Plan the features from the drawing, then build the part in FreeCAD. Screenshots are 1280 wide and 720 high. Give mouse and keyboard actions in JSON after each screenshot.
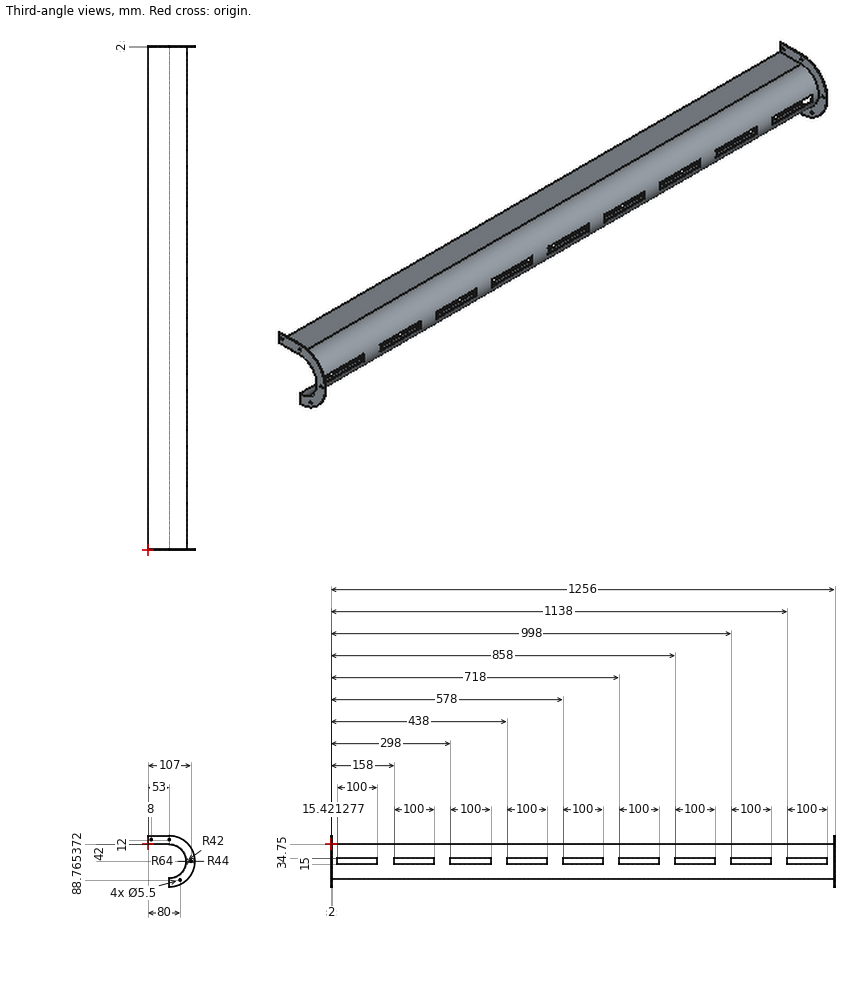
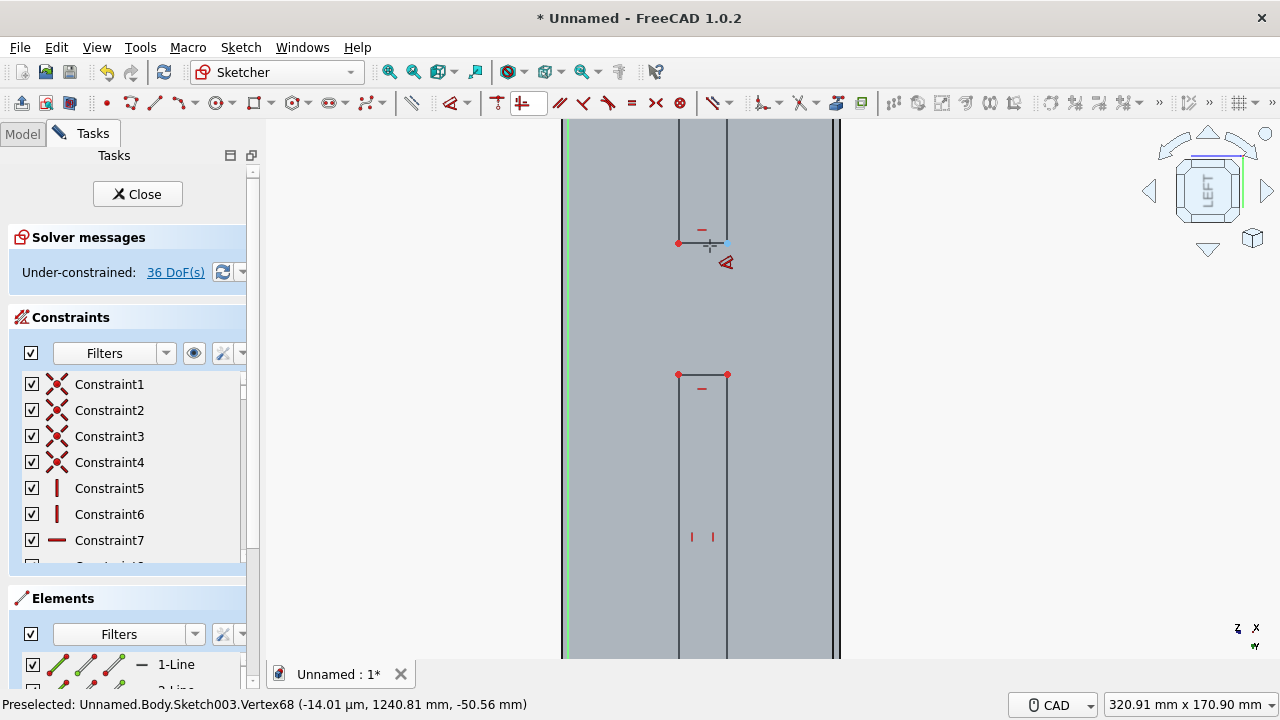
{"action": "left_click", "coordinate": [703, 243]}
{"action": "left_click", "coordinate": [703, 209]}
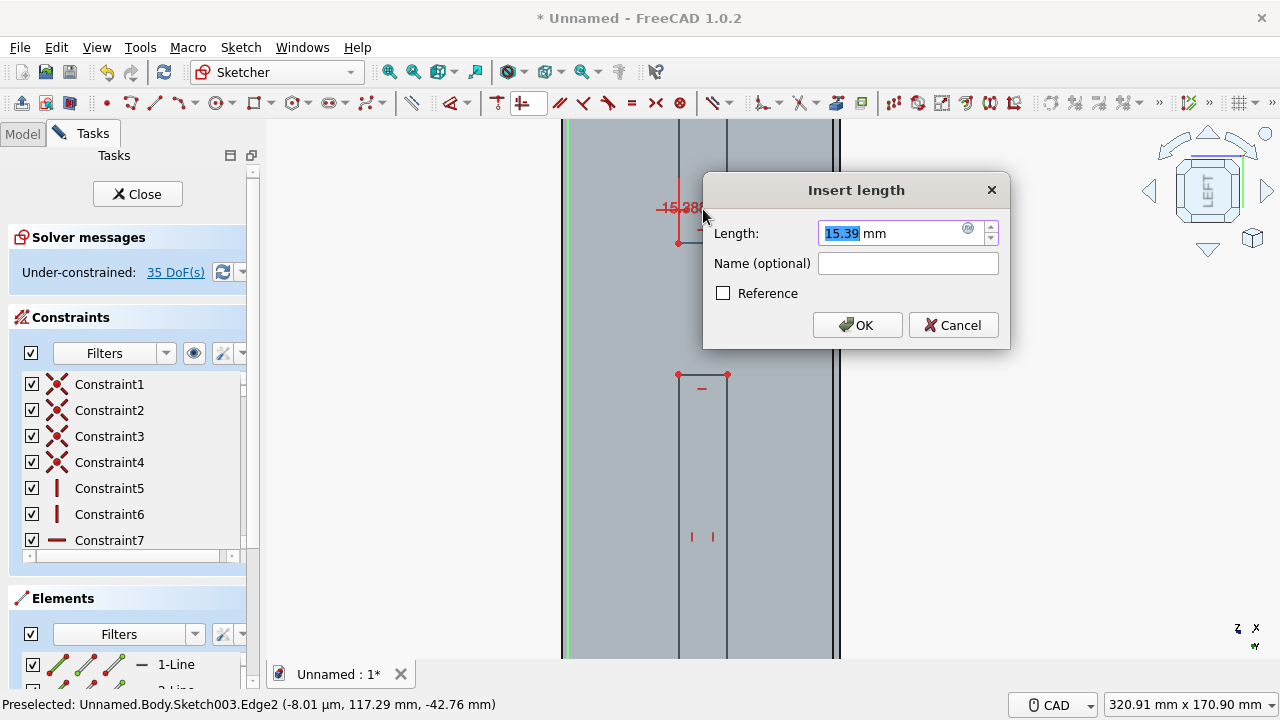
{"action": "type", "text": "15"}
{"action": "key", "text": "Return"}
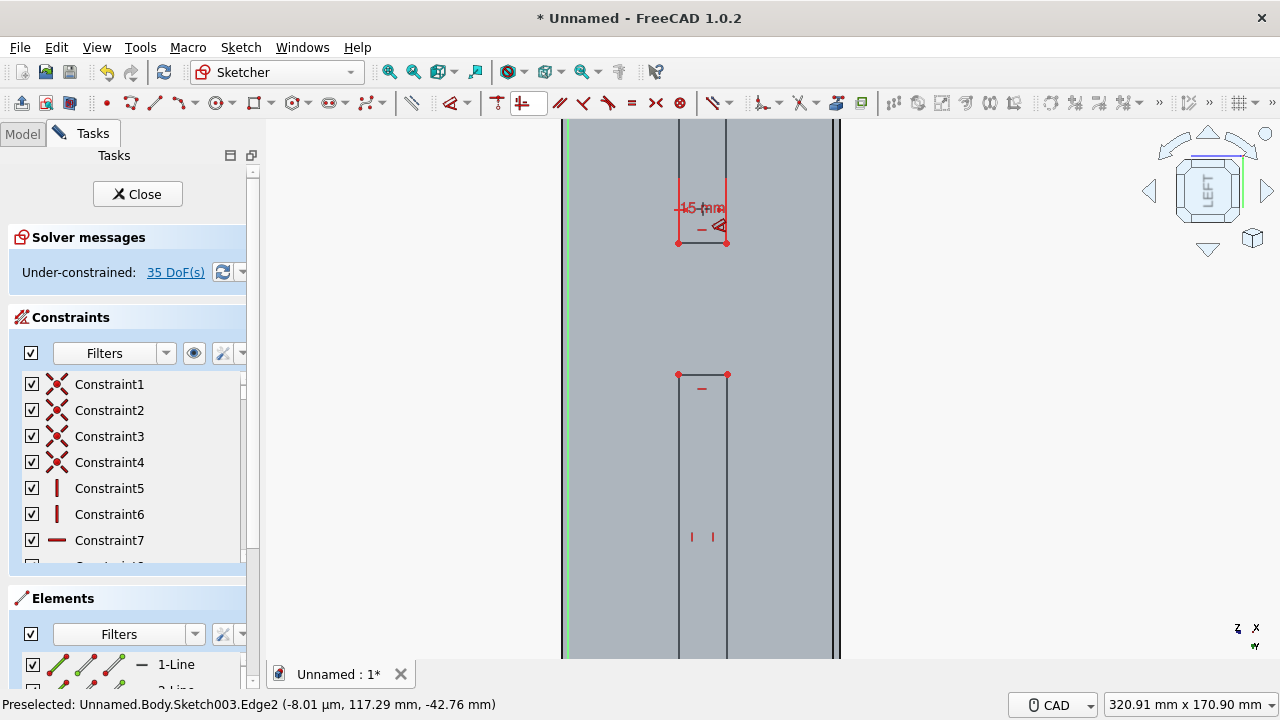
{"action": "scroll", "coordinate": [710, 245], "scroll_direction": "down", "scroll_amount": 12}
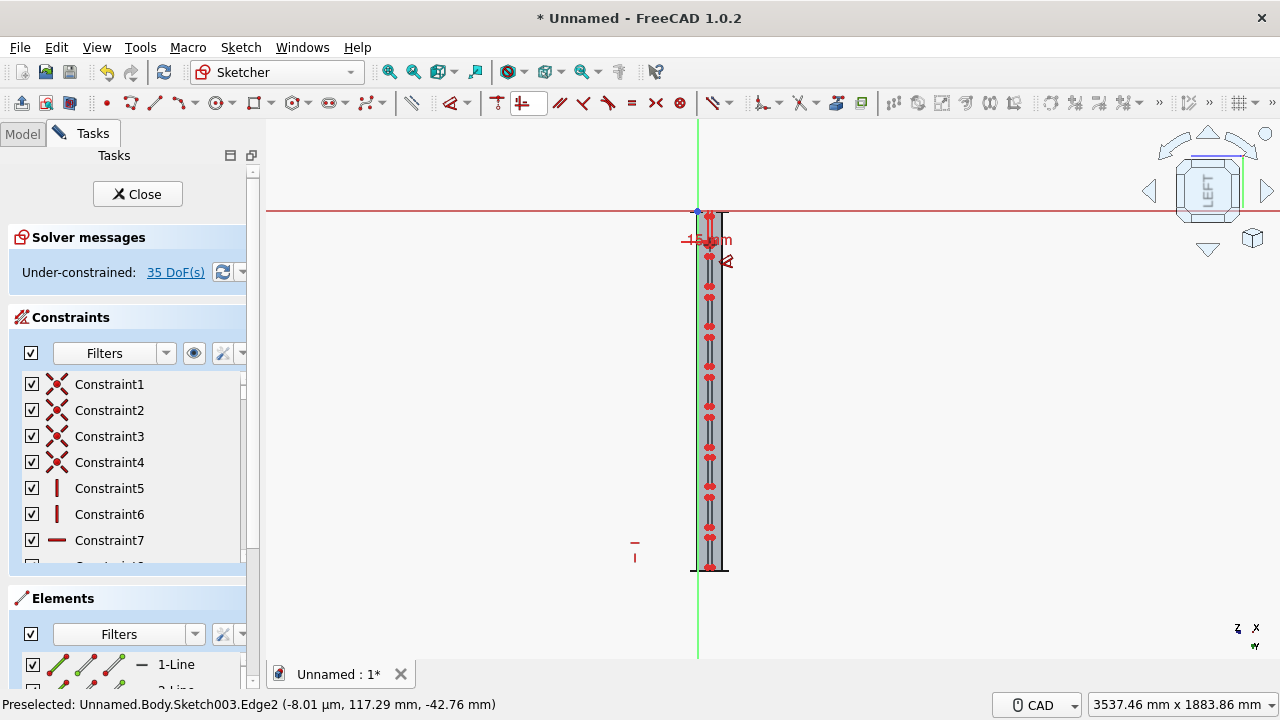
{"action": "scroll", "coordinate": [709, 286], "scroll_direction": "up", "scroll_amount": 12}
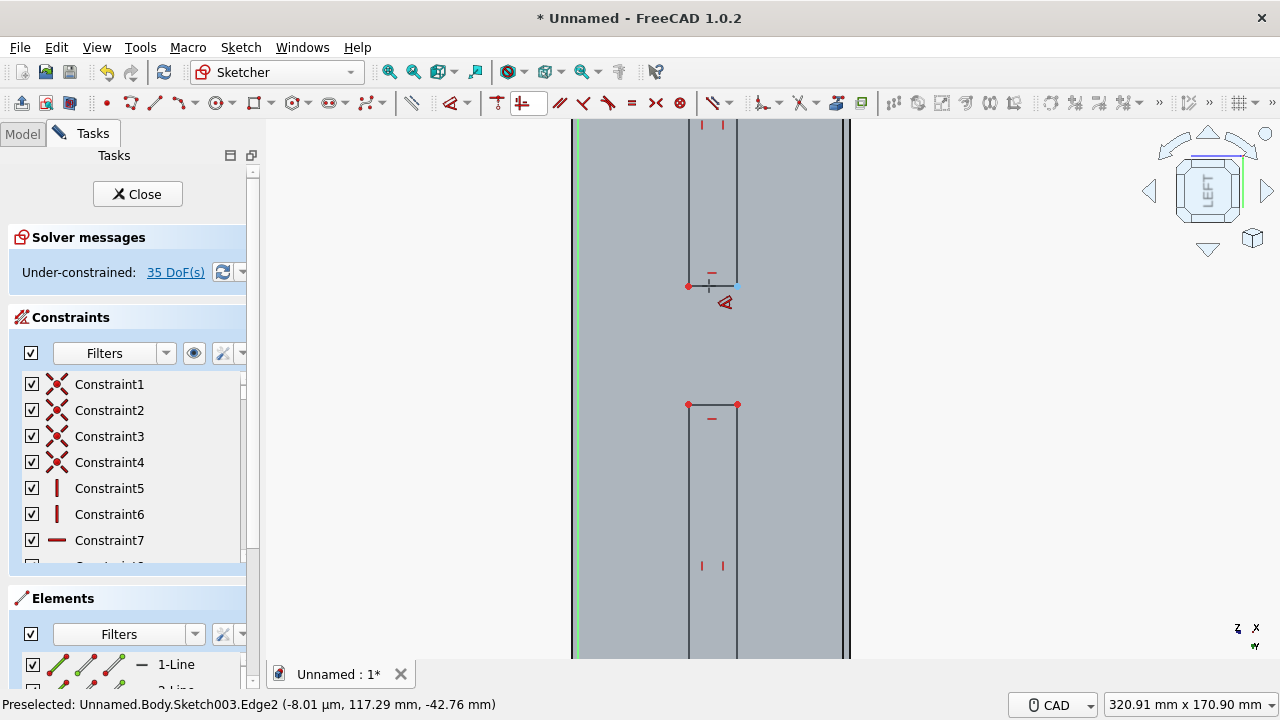
{"action": "left_click", "coordinate": [703, 286]}
{"action": "left_click", "coordinate": [713, 252]}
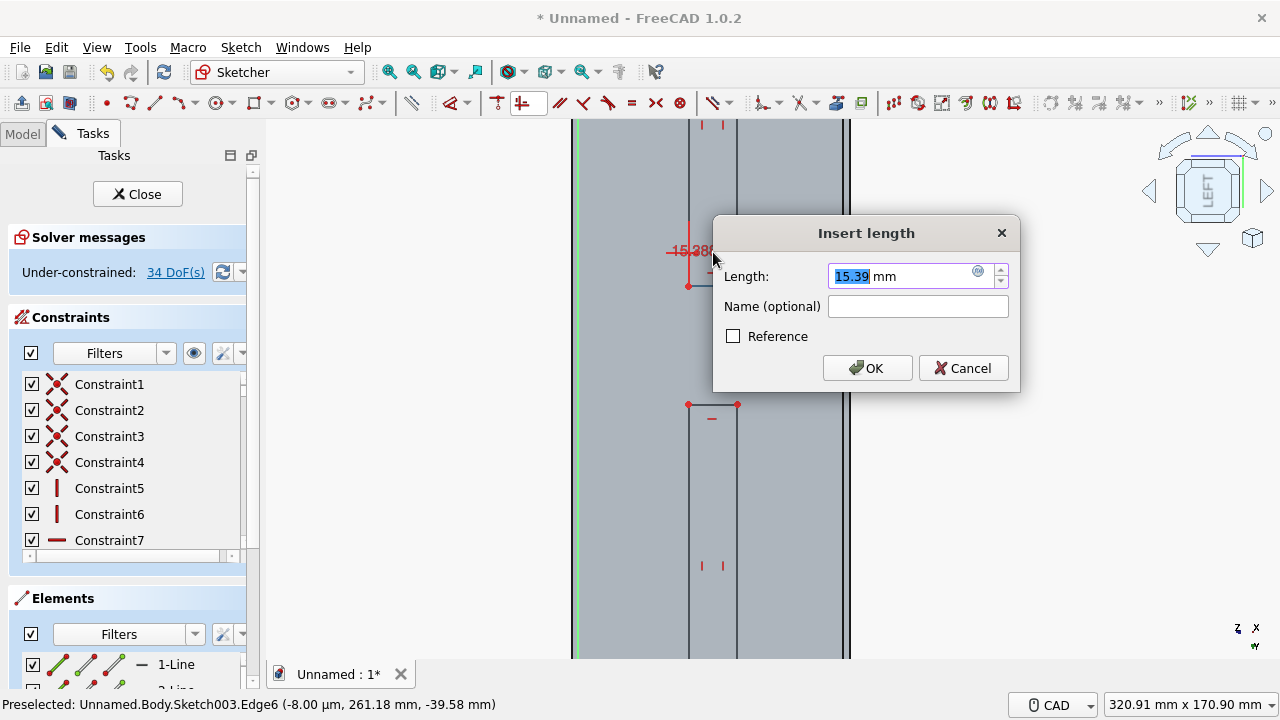
{"action": "type", "text": "15"}
{"action": "key", "text": "Return"}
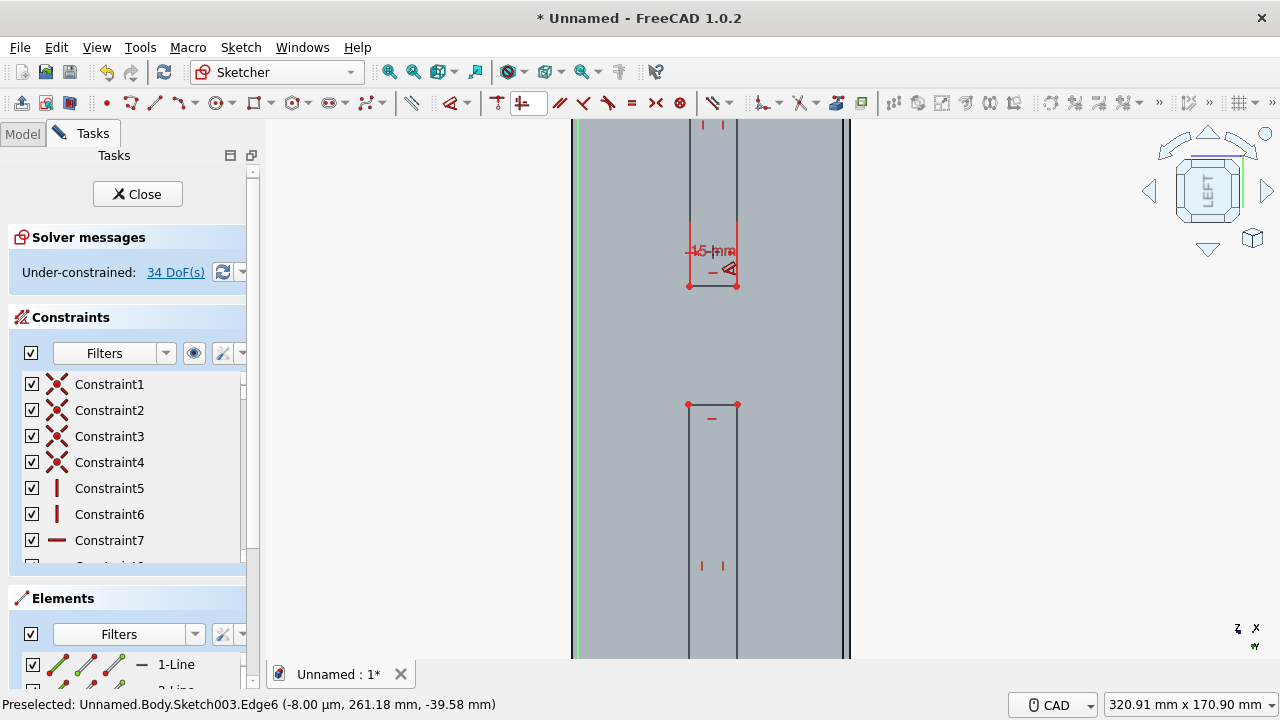
{"action": "scroll", "coordinate": [709, 286], "scroll_direction": "down", "scroll_amount": 12}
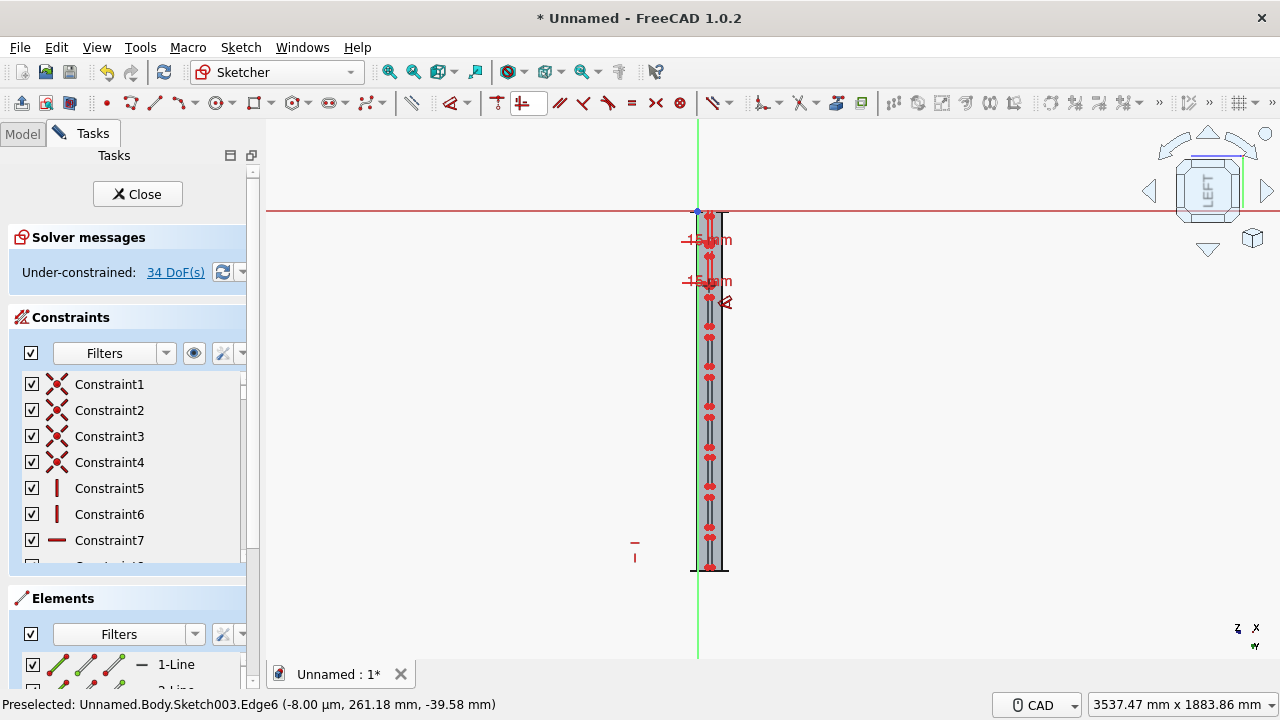
{"action": "scroll", "coordinate": [709, 527], "scroll_direction": "up", "scroll_amount": 12}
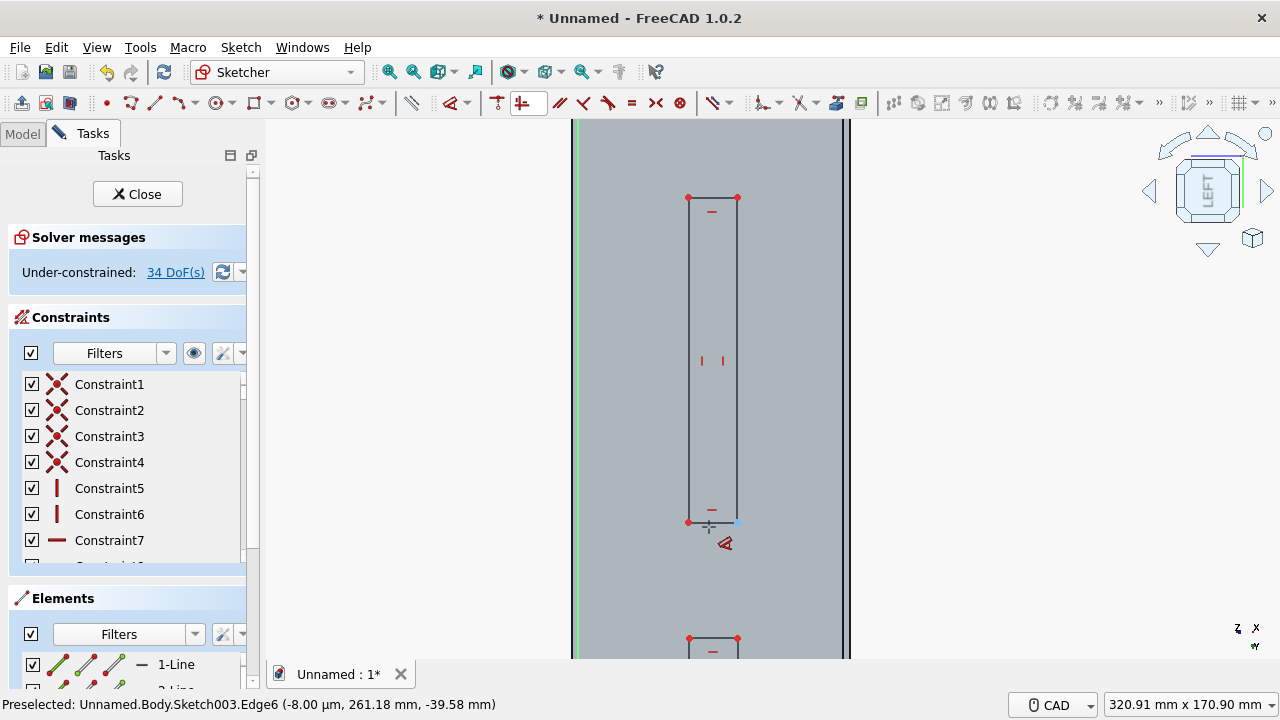
{"action": "left_click", "coordinate": [703, 523]}
{"action": "left_click", "coordinate": [713, 557]}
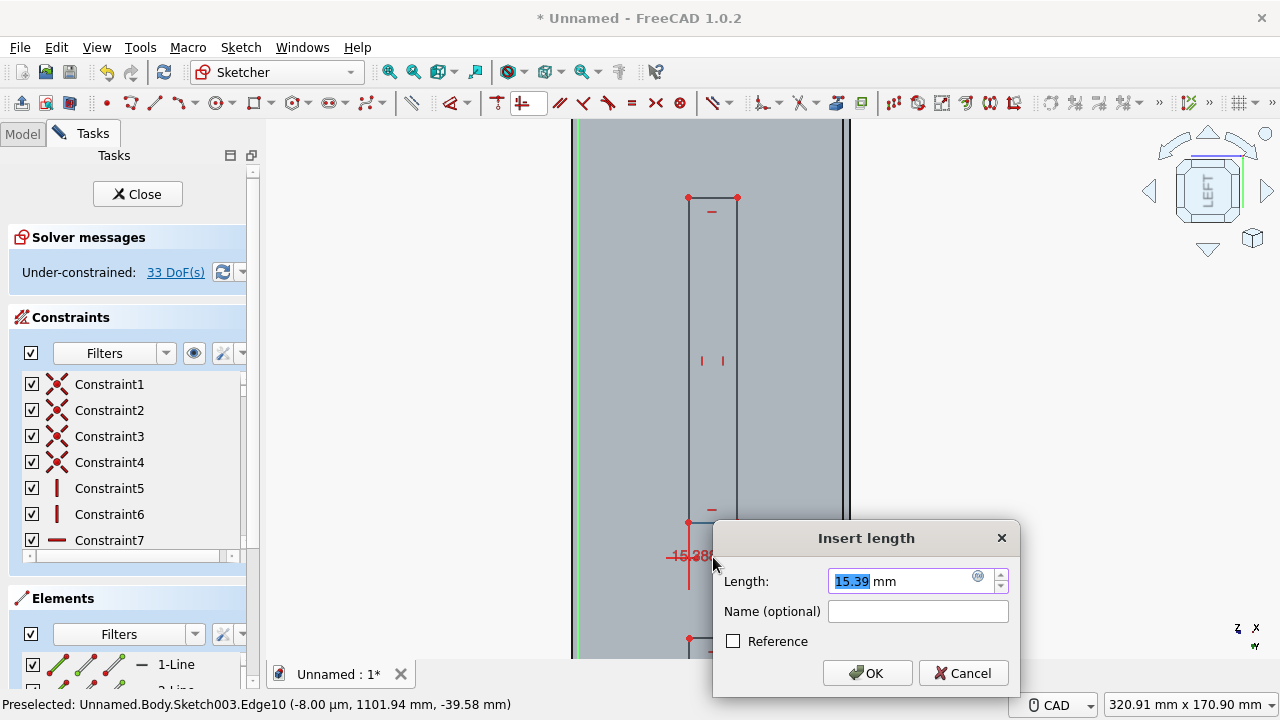
{"action": "type", "text": "15"}
{"action": "key", "text": "Return"}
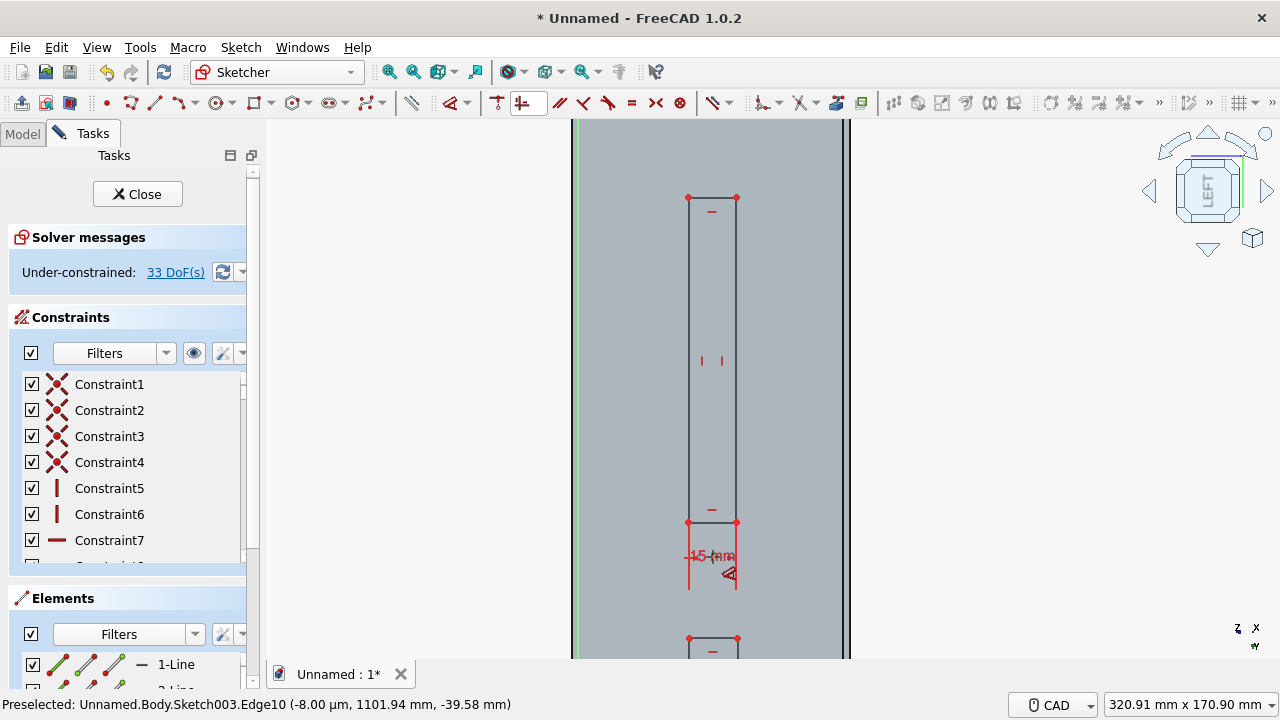
{"action": "scroll", "coordinate": [709, 528], "scroll_direction": "down", "scroll_amount": 12}